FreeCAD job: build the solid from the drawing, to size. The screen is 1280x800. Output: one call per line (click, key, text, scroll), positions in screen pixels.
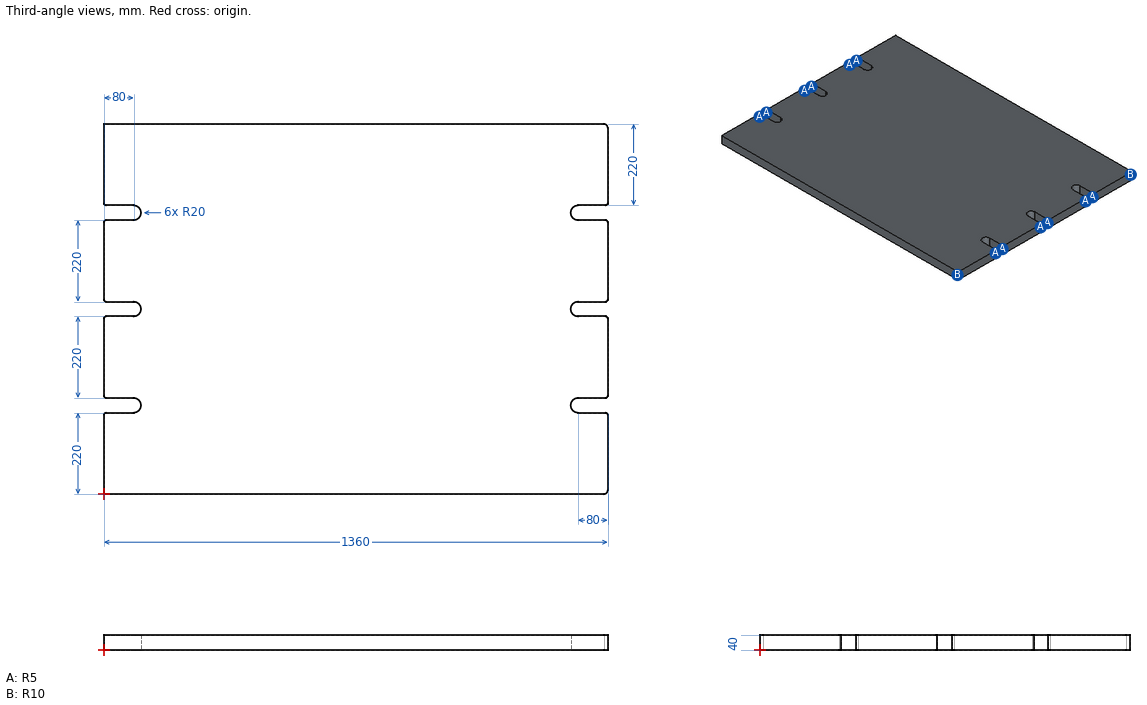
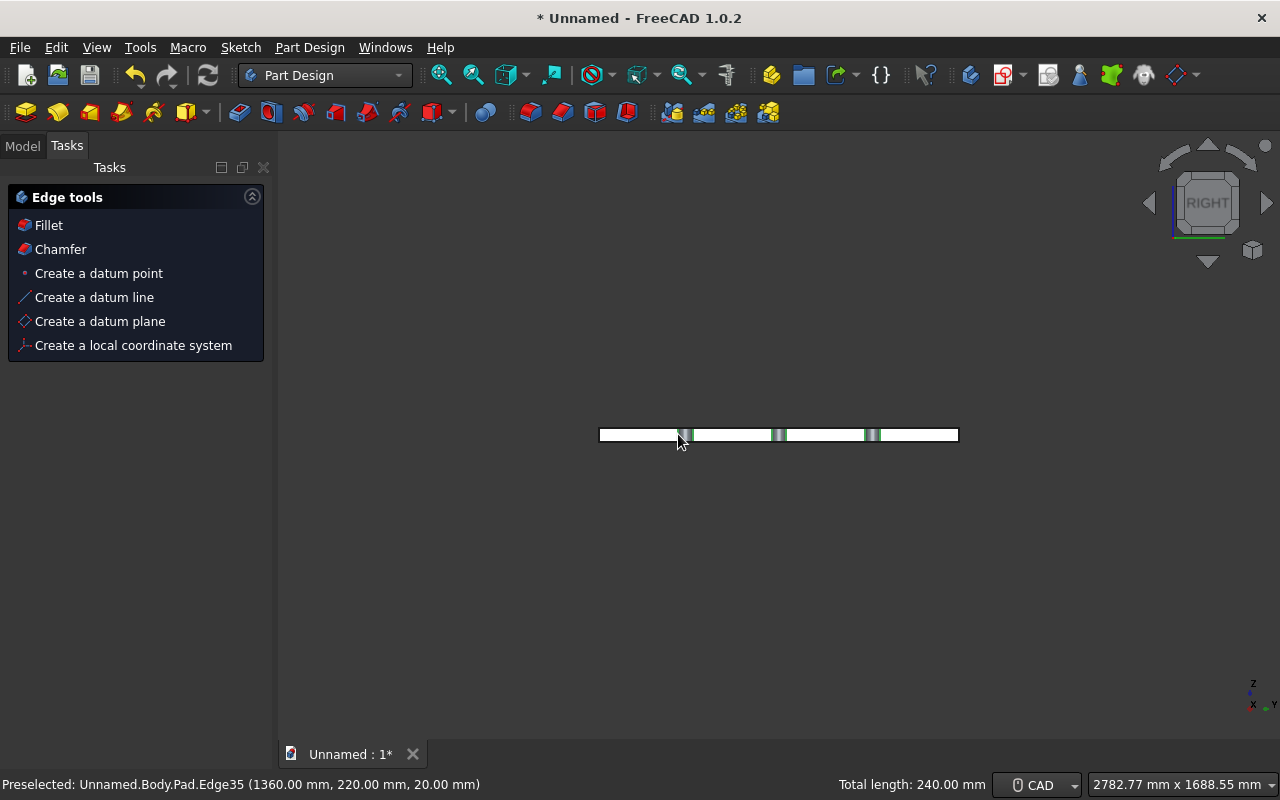
scroll(678, 434, up, 6)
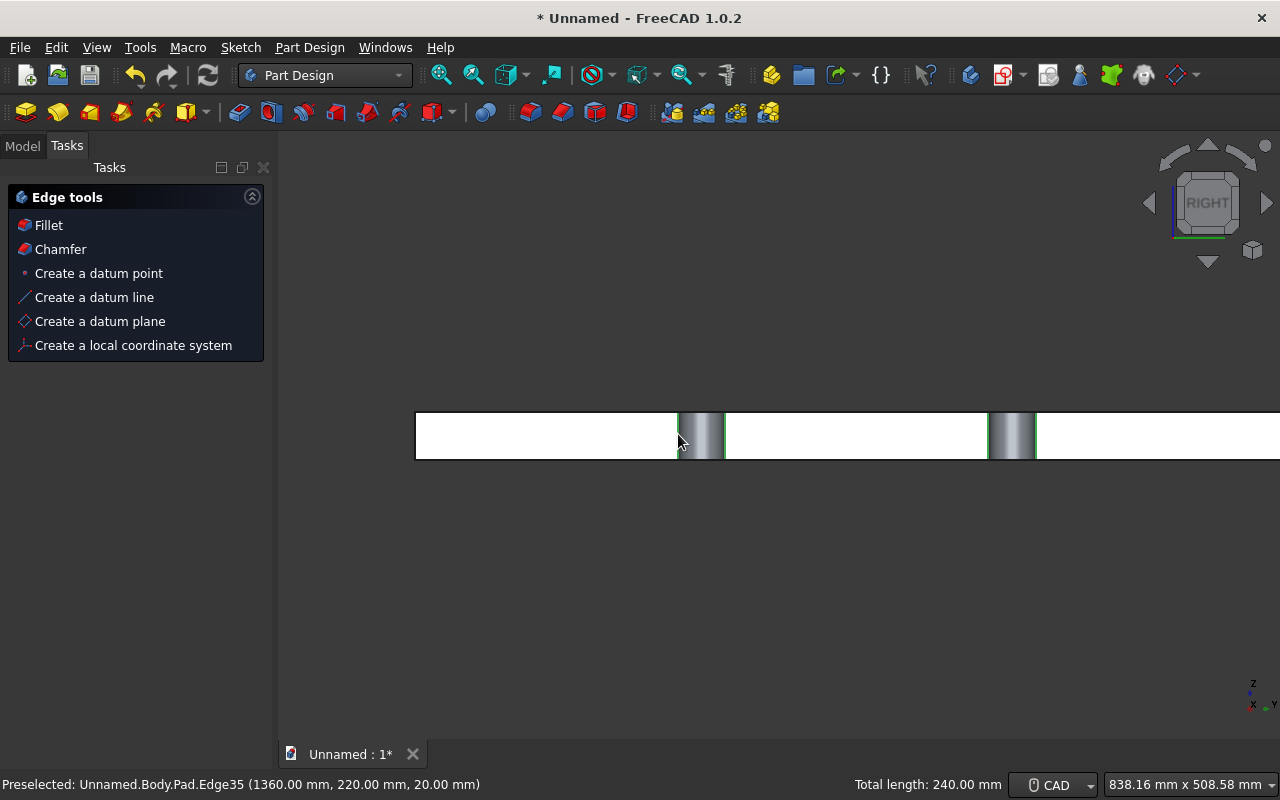
click(442, 76)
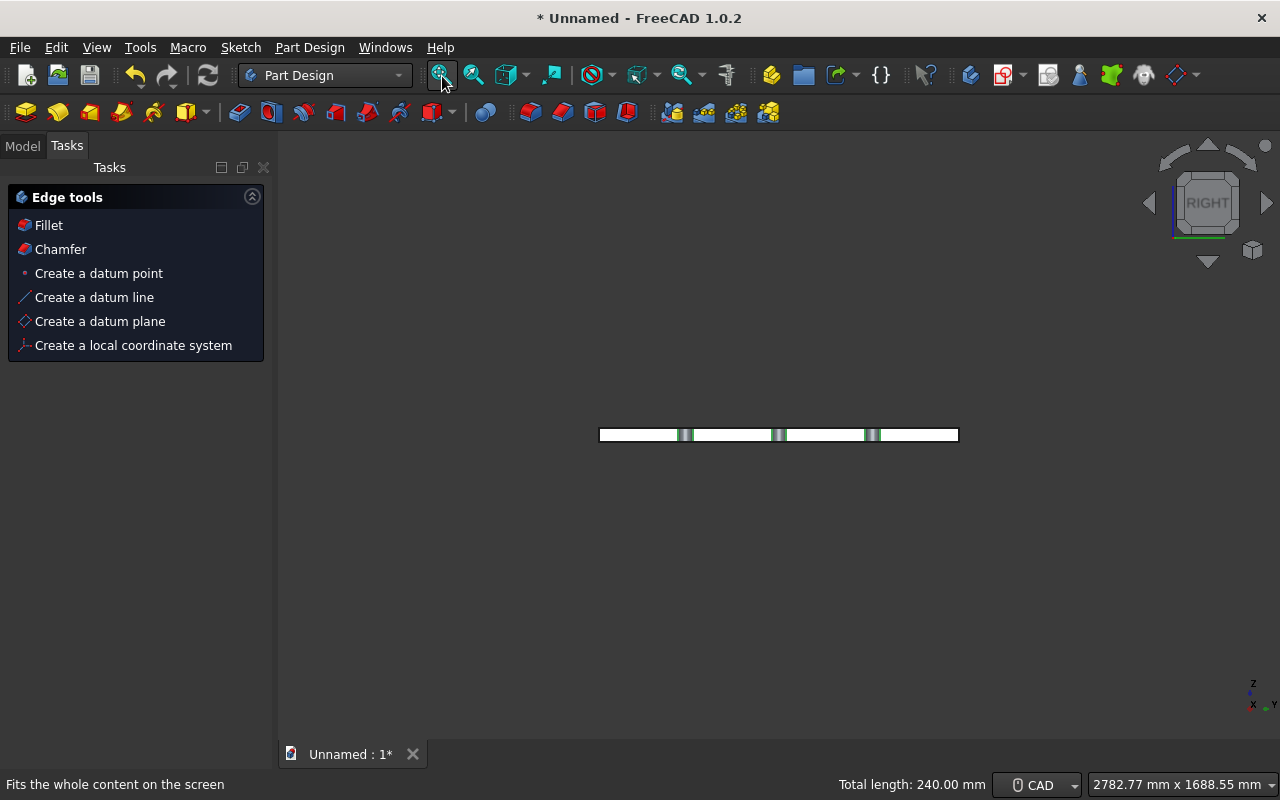
key(5)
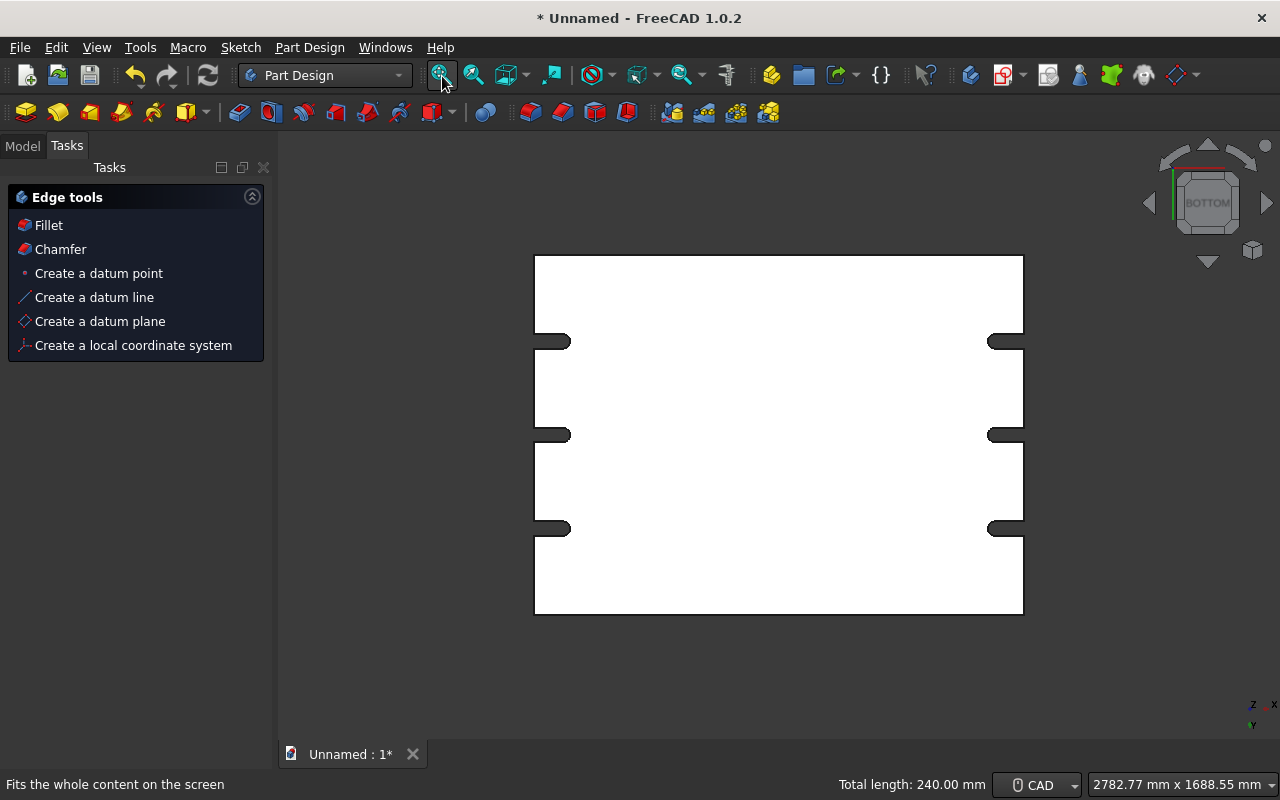
scroll(534, 333, up, 6)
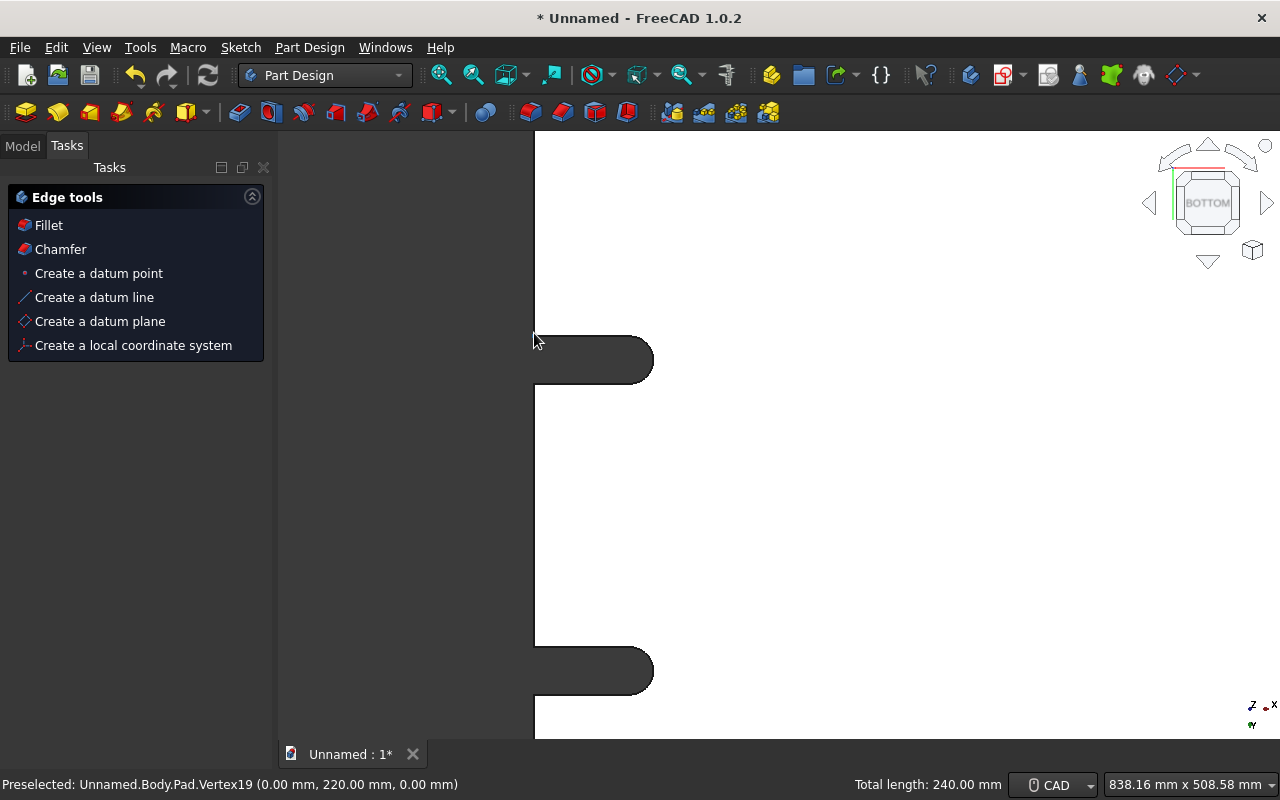
click(442, 76)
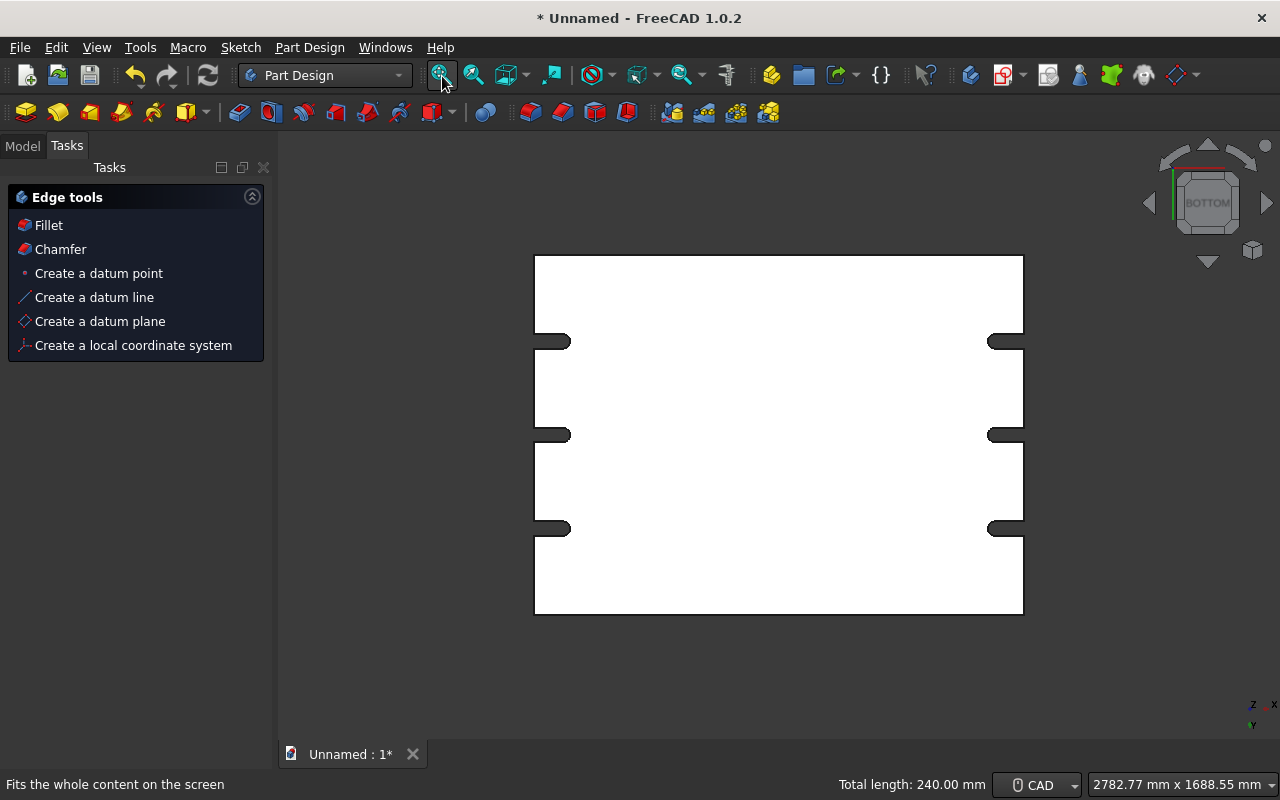
key(4)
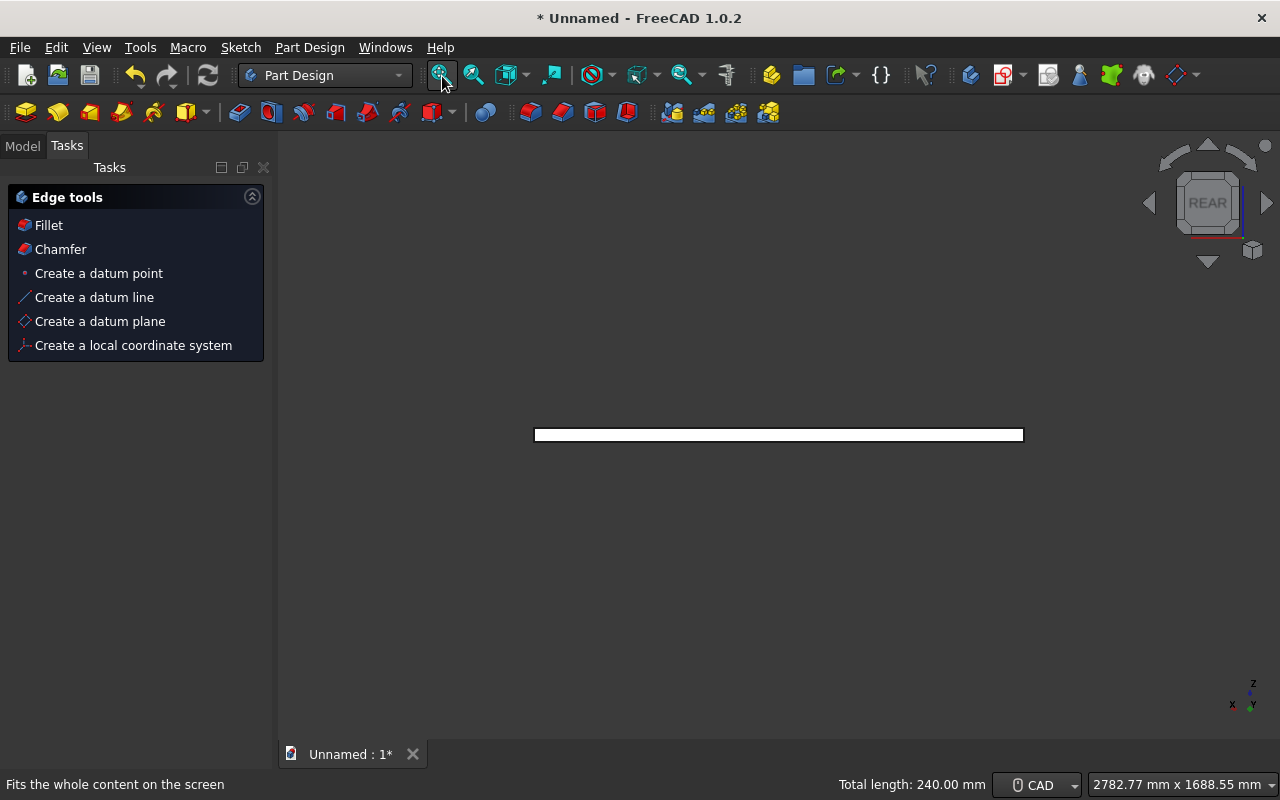
scroll(1024, 434, up, 6)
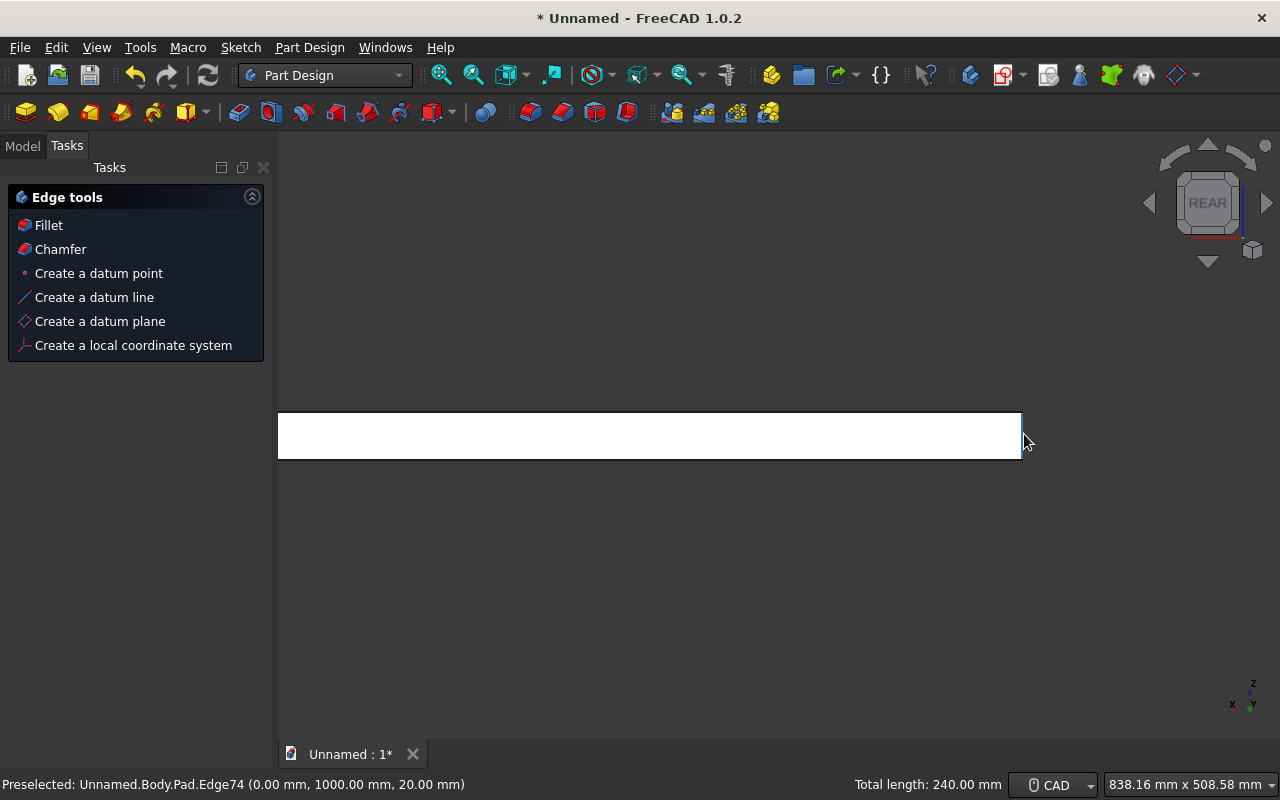
click(442, 76)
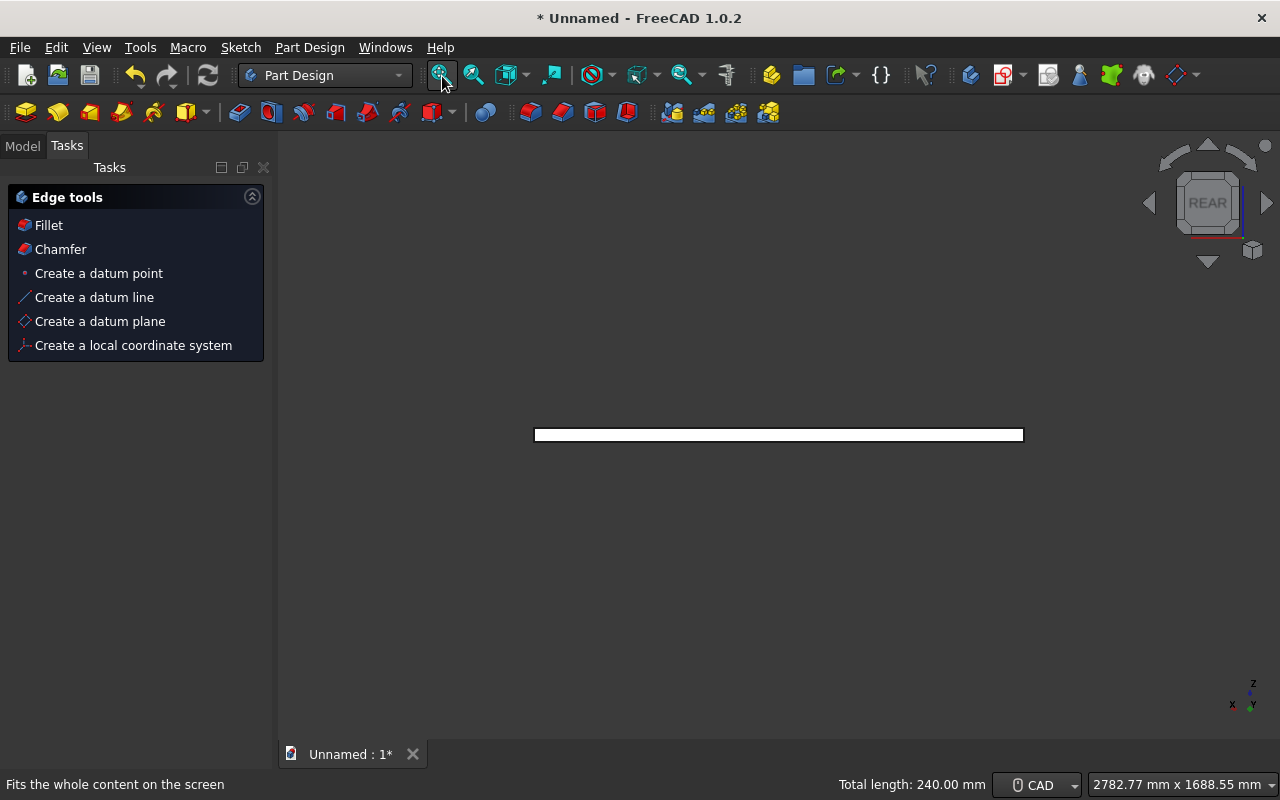
key(6)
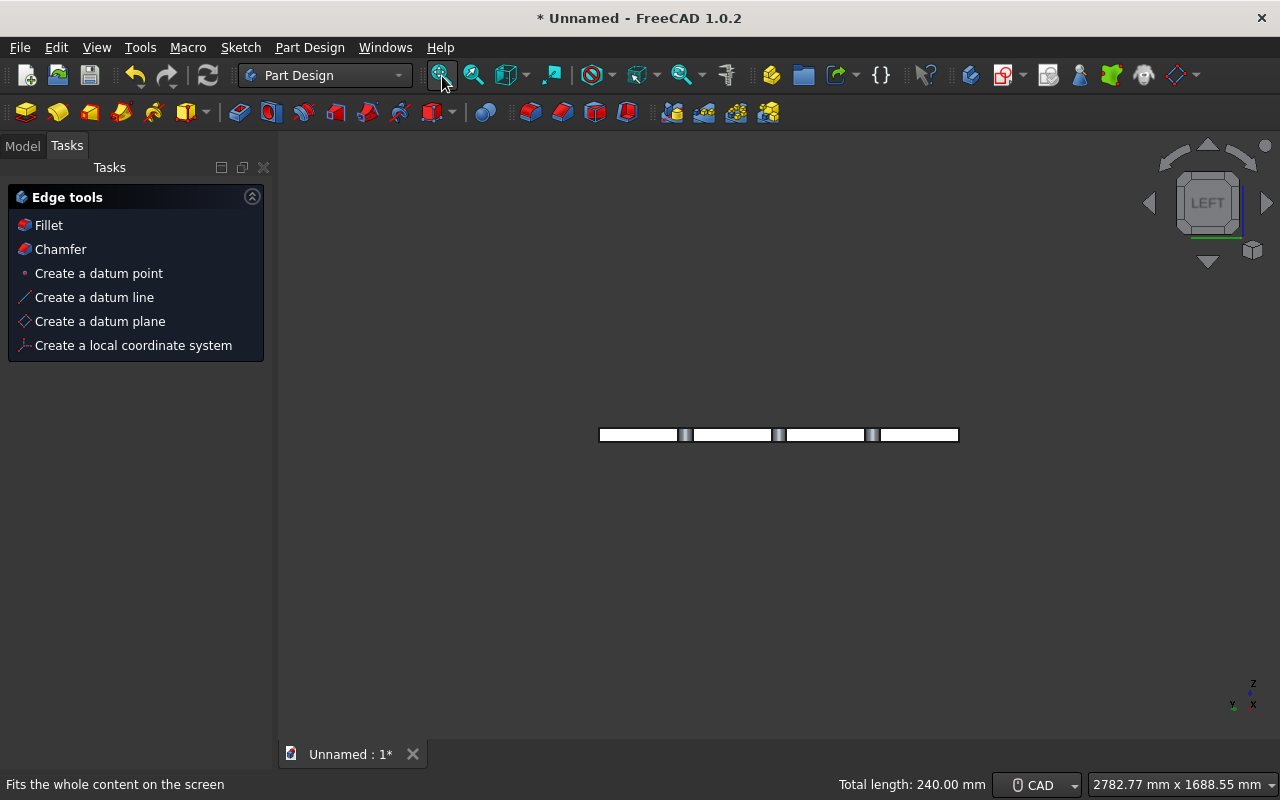
click(442, 76)